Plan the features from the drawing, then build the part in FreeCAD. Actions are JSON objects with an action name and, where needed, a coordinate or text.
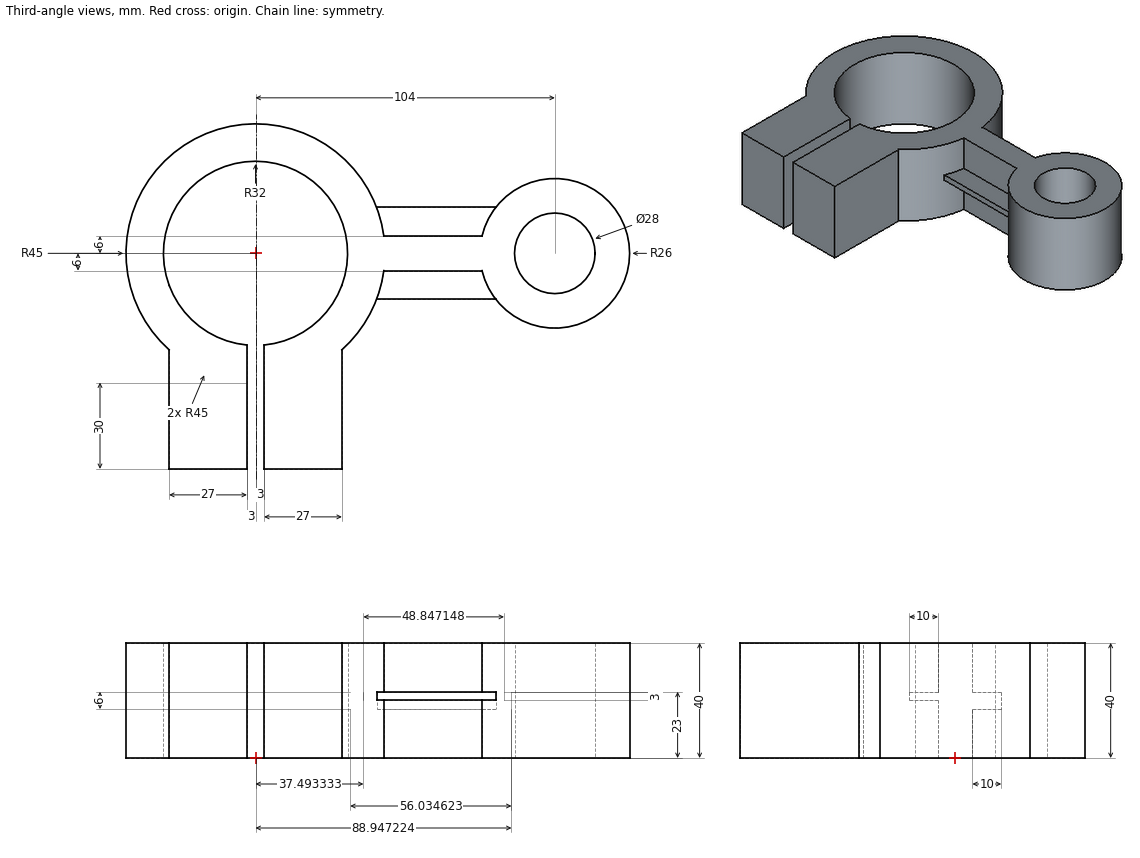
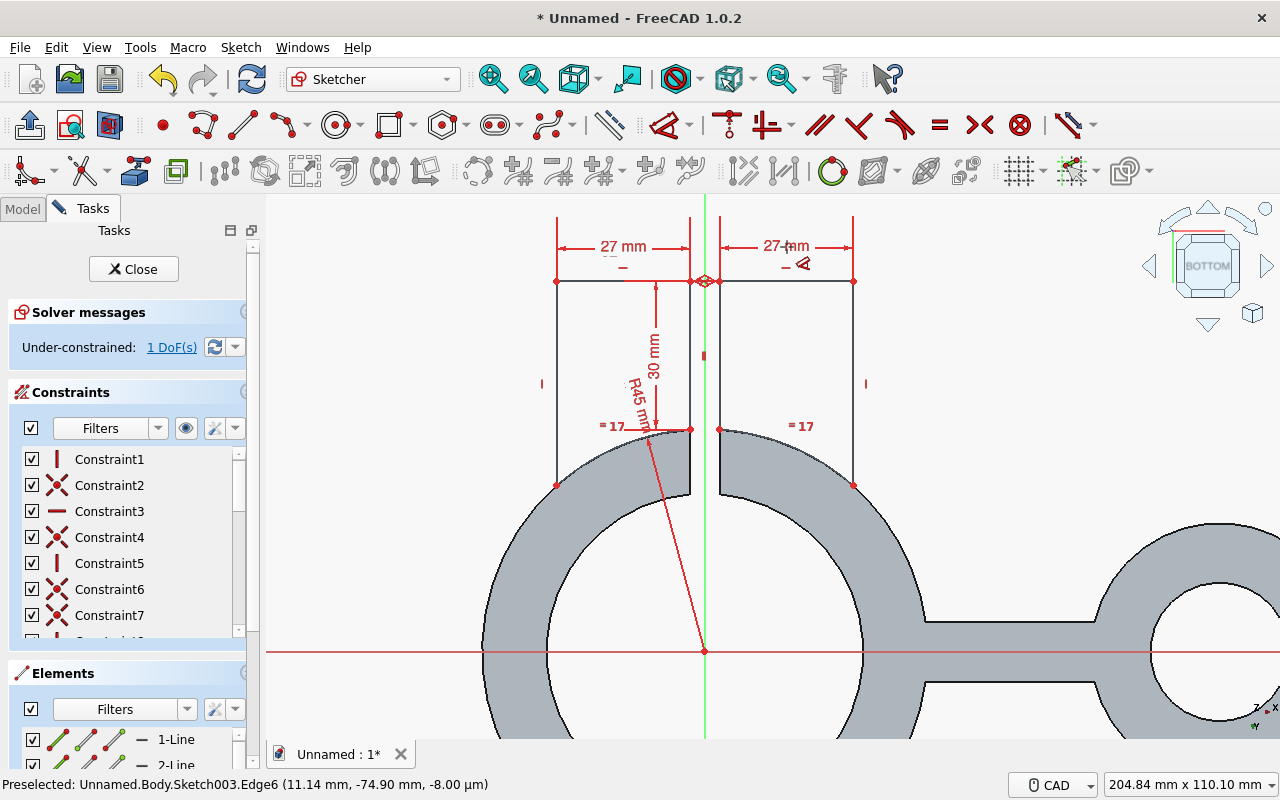
{"action": "scroll", "coordinate": [690, 281], "scroll_direction": "up", "scroll_amount": 5}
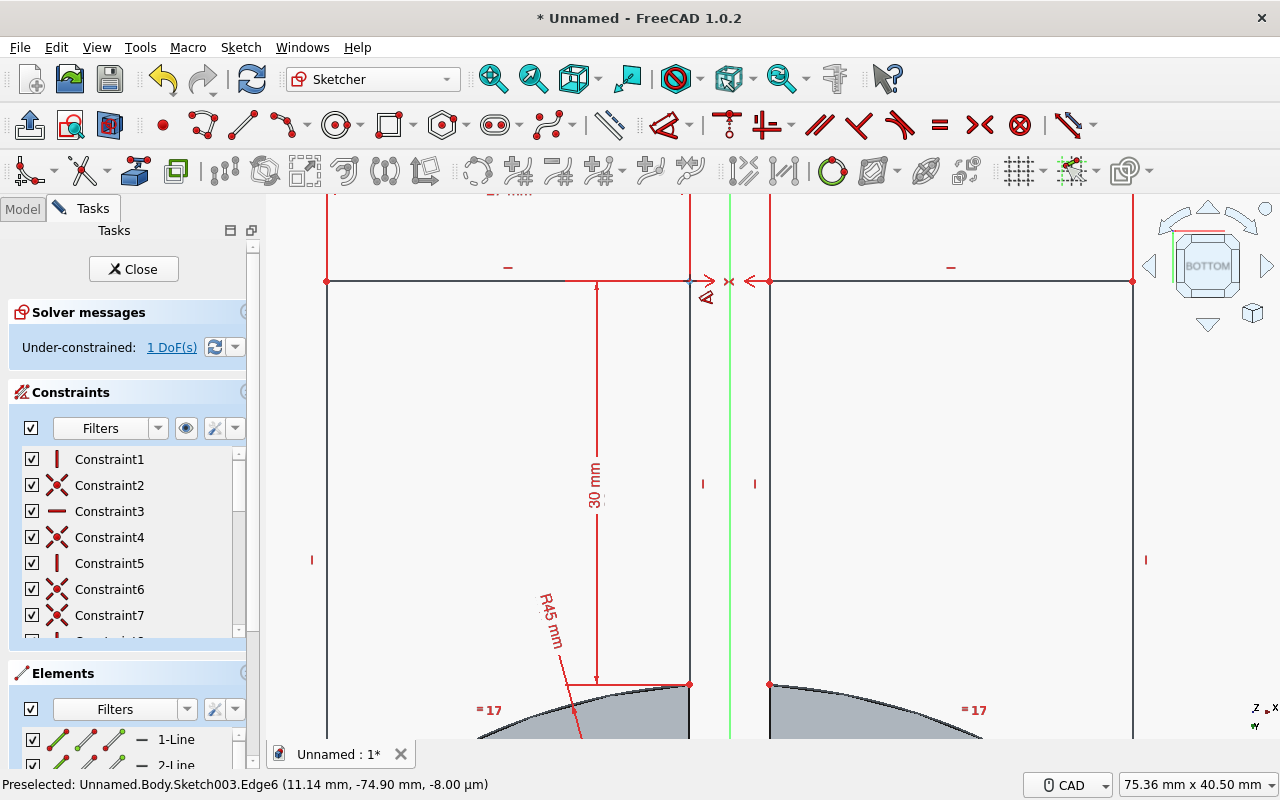
{"action": "left_click", "coordinate": [690, 281]}
{"action": "left_click", "coordinate": [710, 247]}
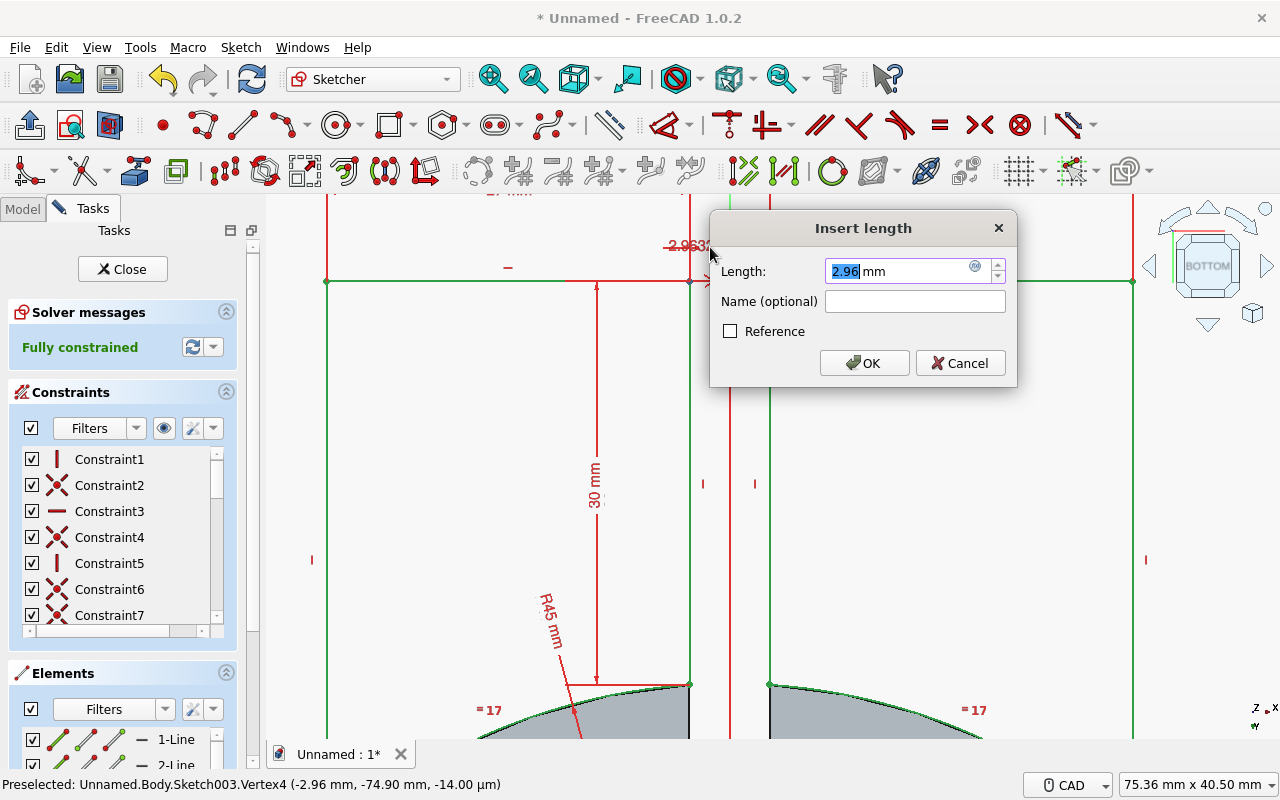
{"action": "type", "text": "3"}
{"action": "key", "text": "Return"}
{"action": "key", "text": "Escape"}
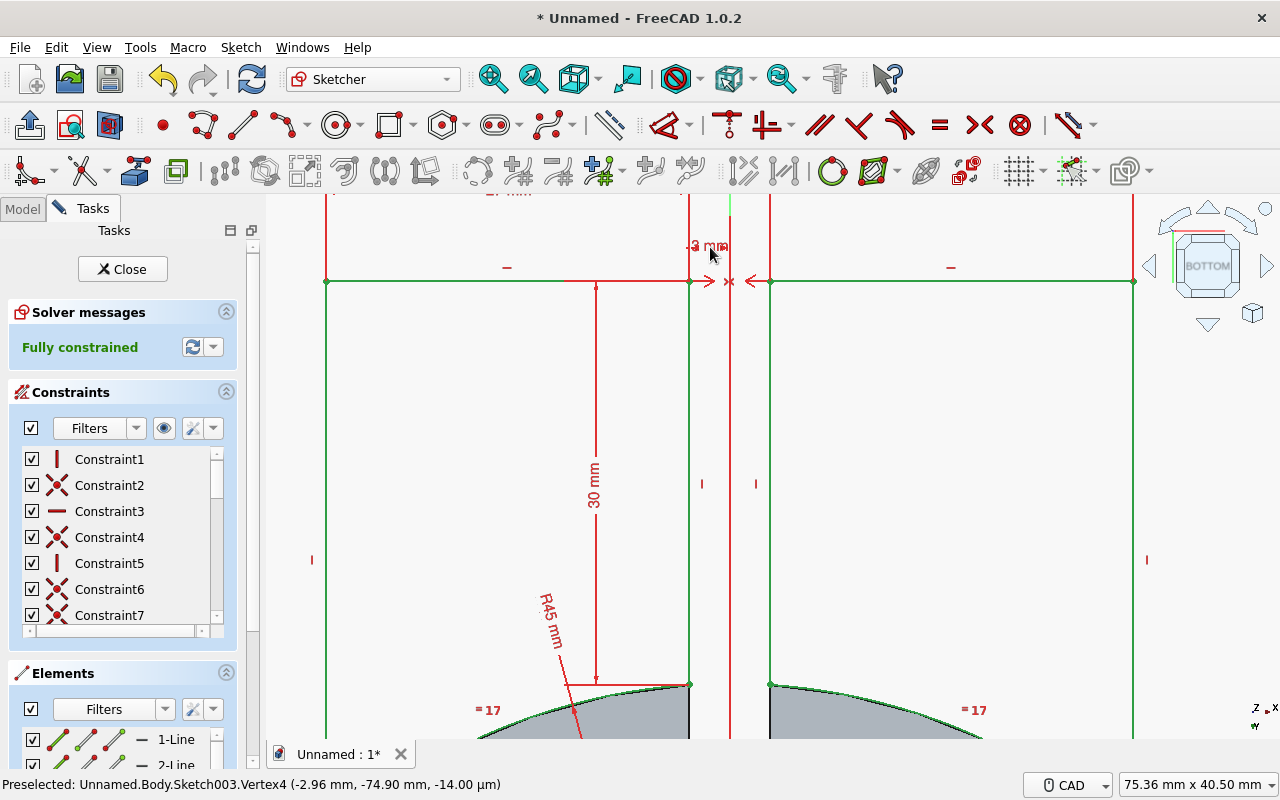
{"action": "left_click", "coordinate": [123, 269]}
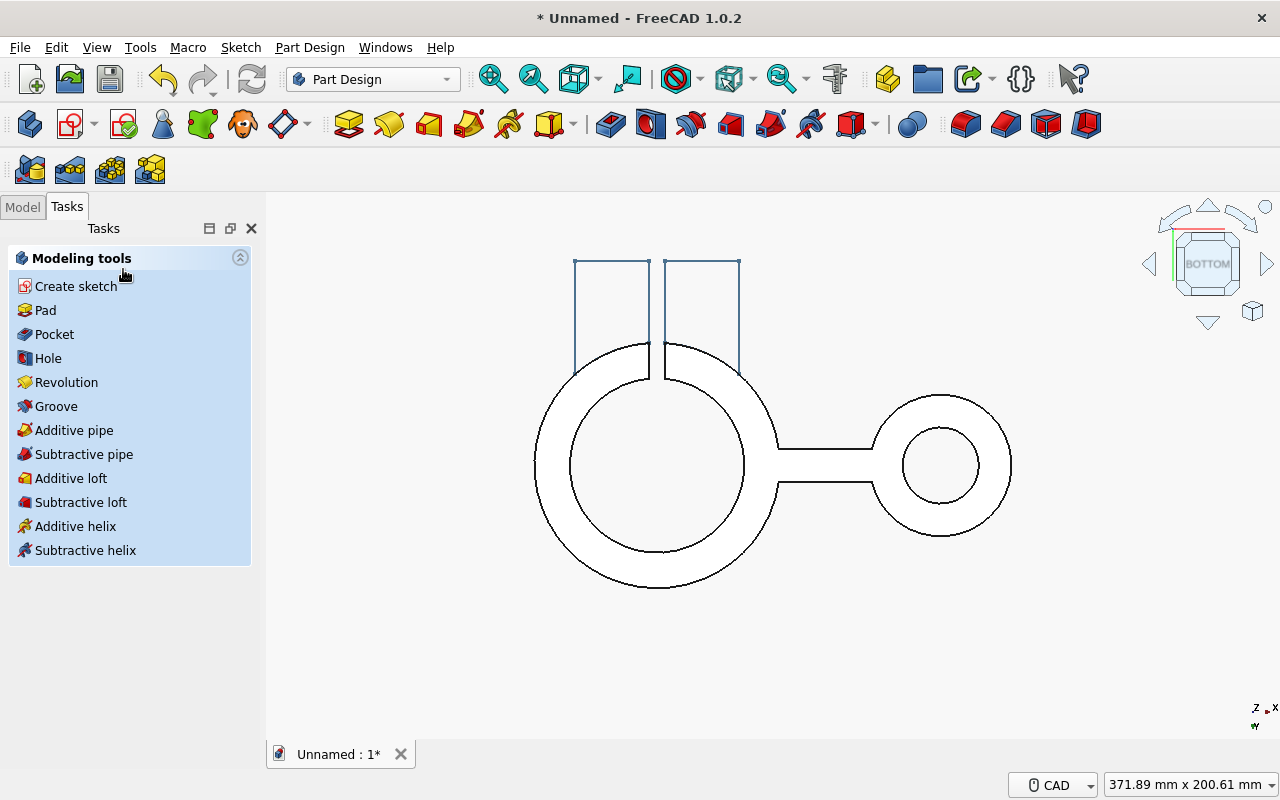
{"action": "left_click", "coordinate": [350, 124]}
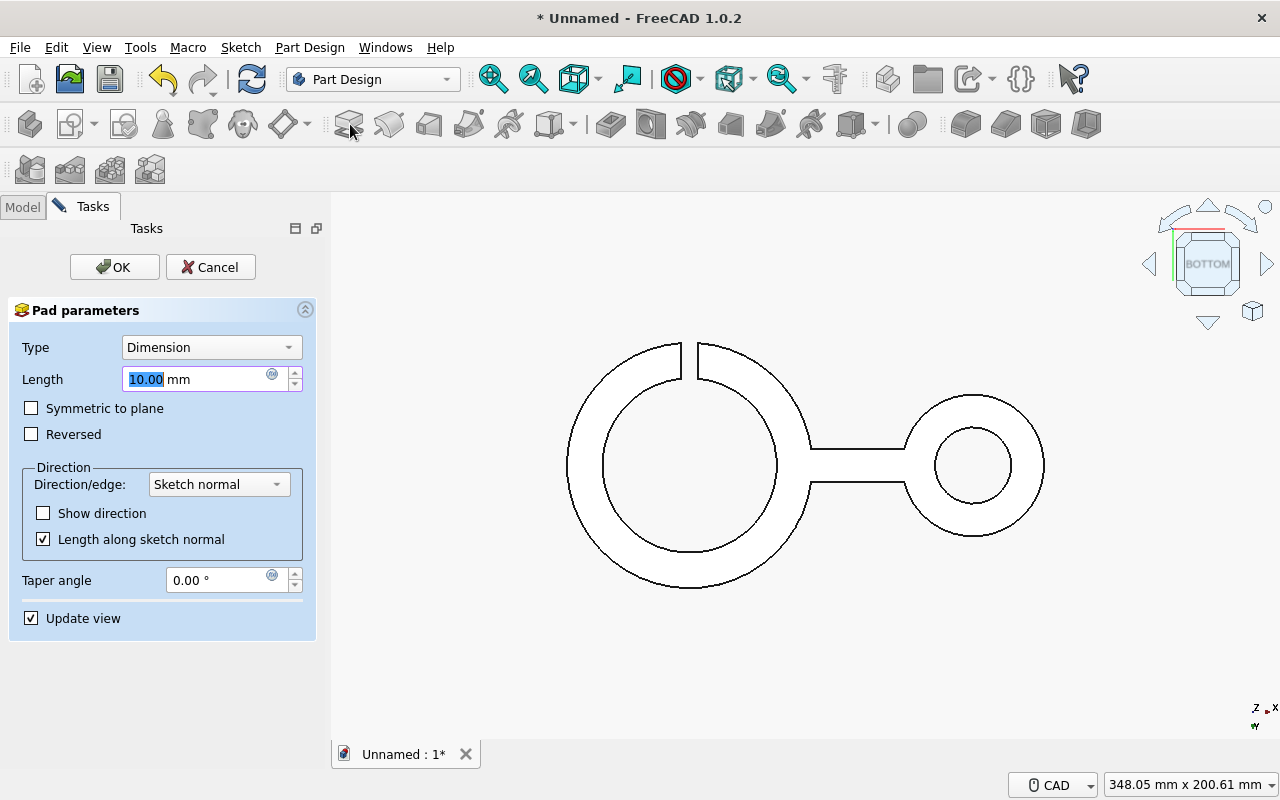
{"action": "type", "text": "40"}
{"action": "key", "text": "Tab"}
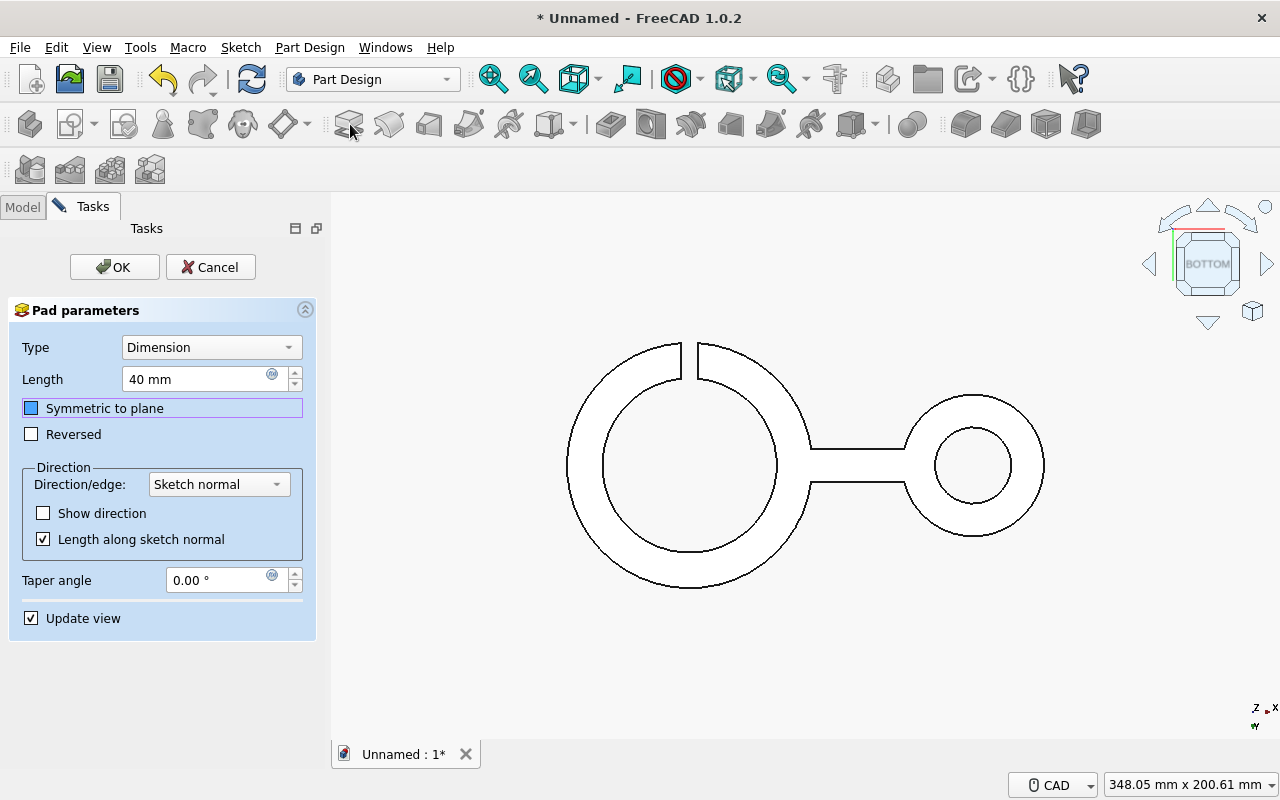
{"action": "left_click", "coordinate": [30, 434]}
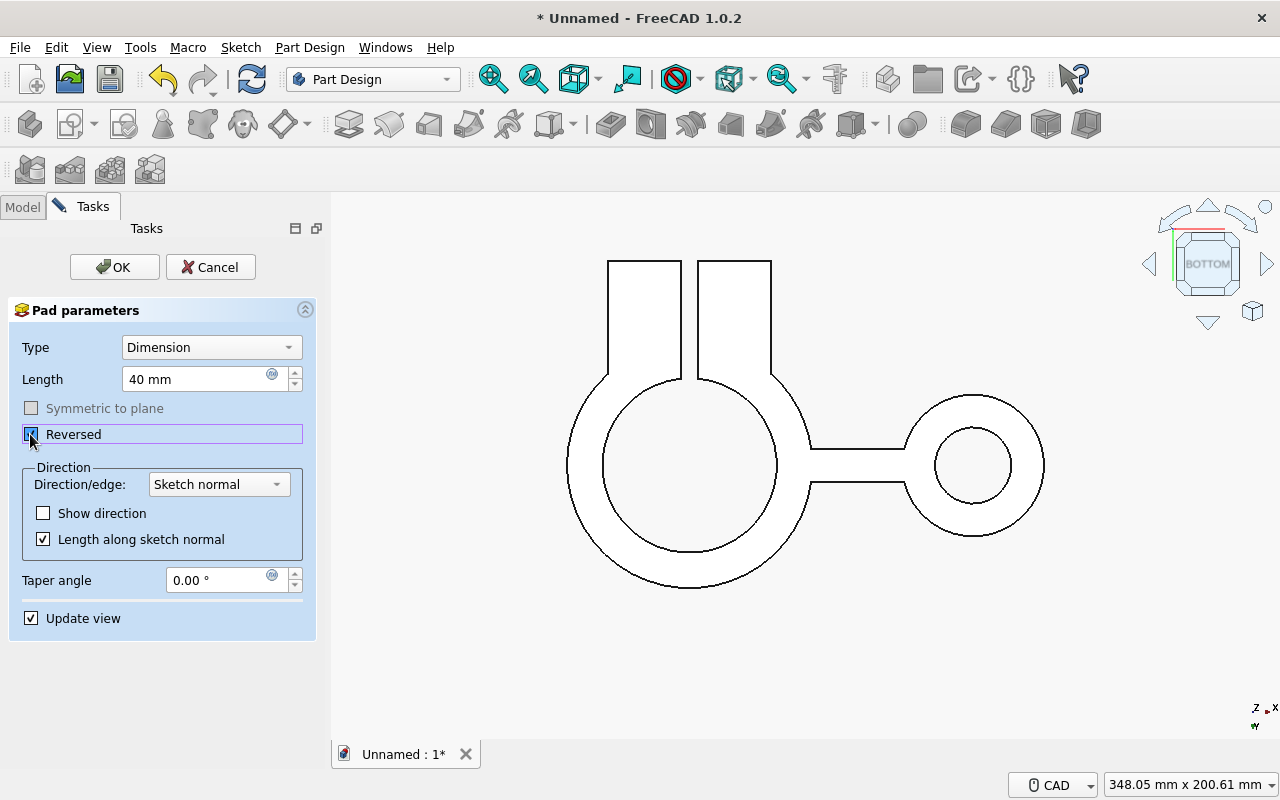
{"action": "left_click", "coordinate": [115, 267]}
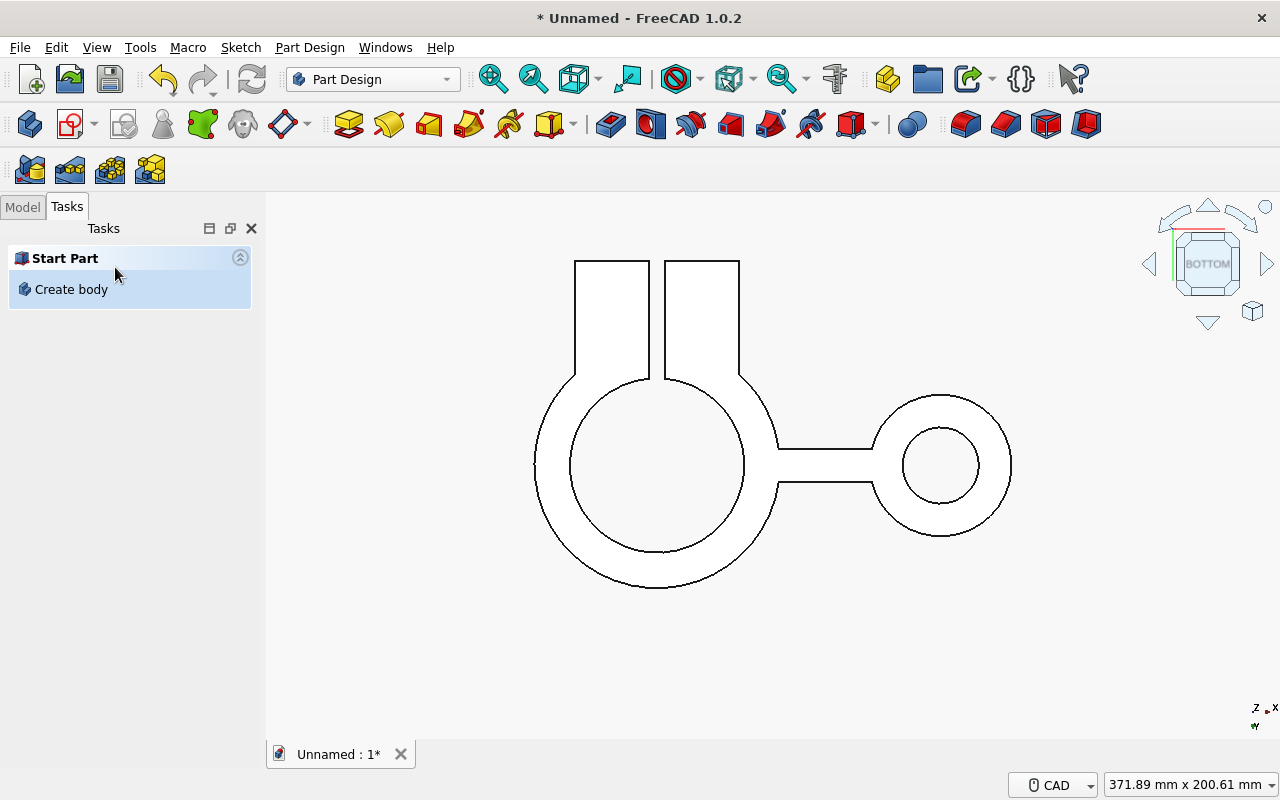
{"action": "key", "text": "4"}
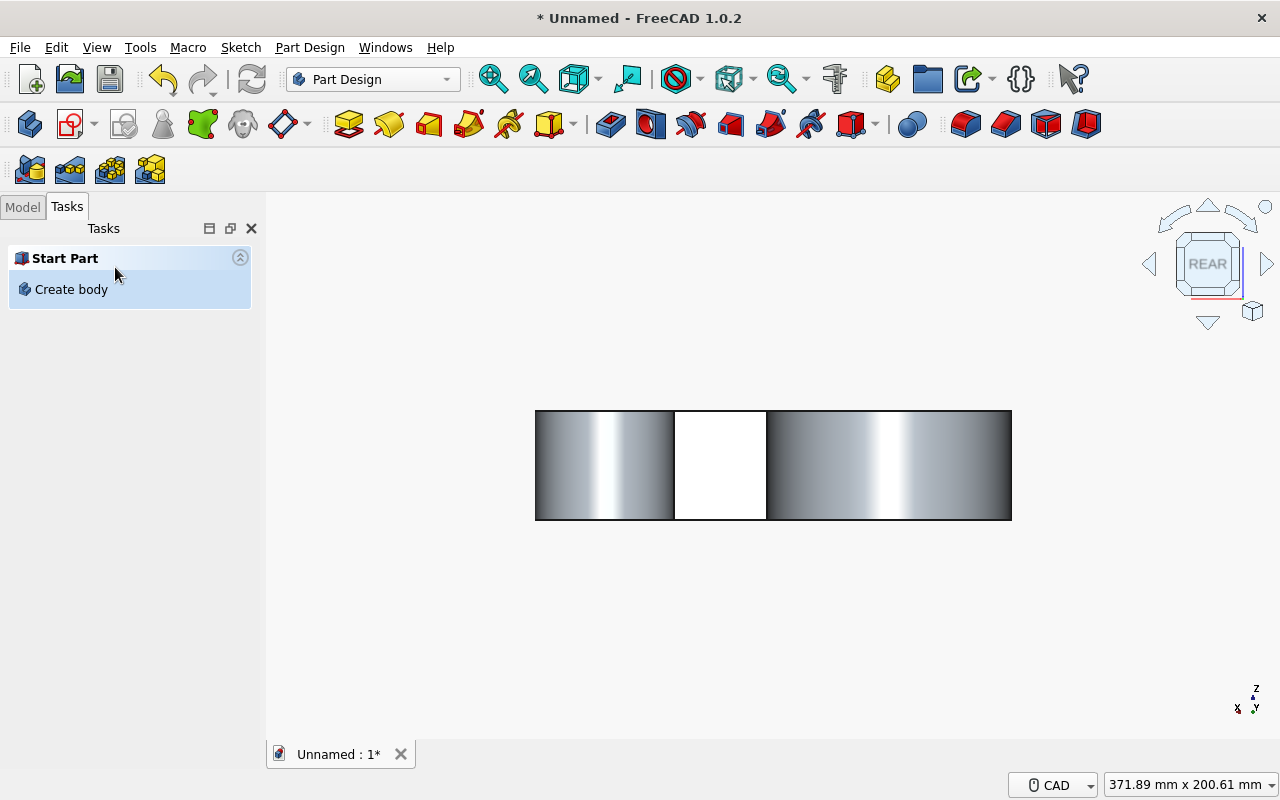
{"action": "left_click", "coordinate": [721, 465]}